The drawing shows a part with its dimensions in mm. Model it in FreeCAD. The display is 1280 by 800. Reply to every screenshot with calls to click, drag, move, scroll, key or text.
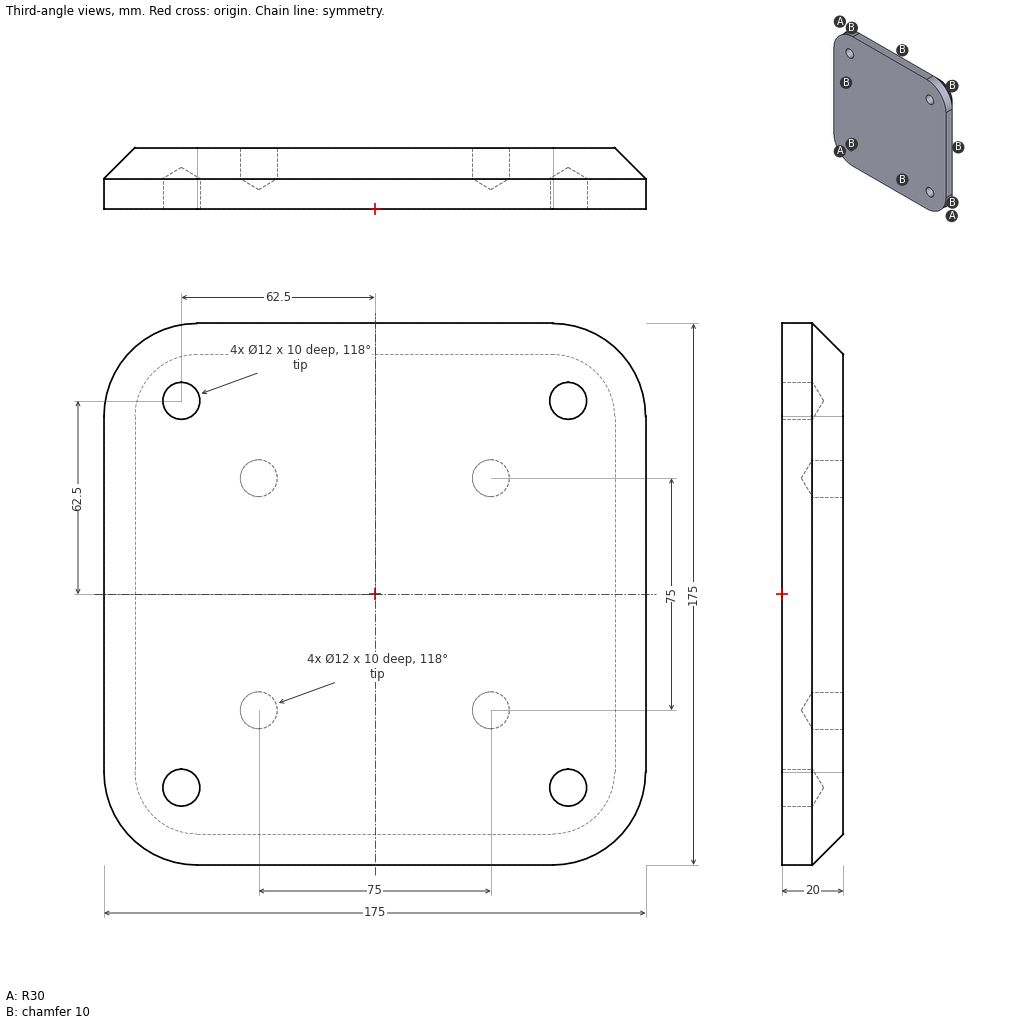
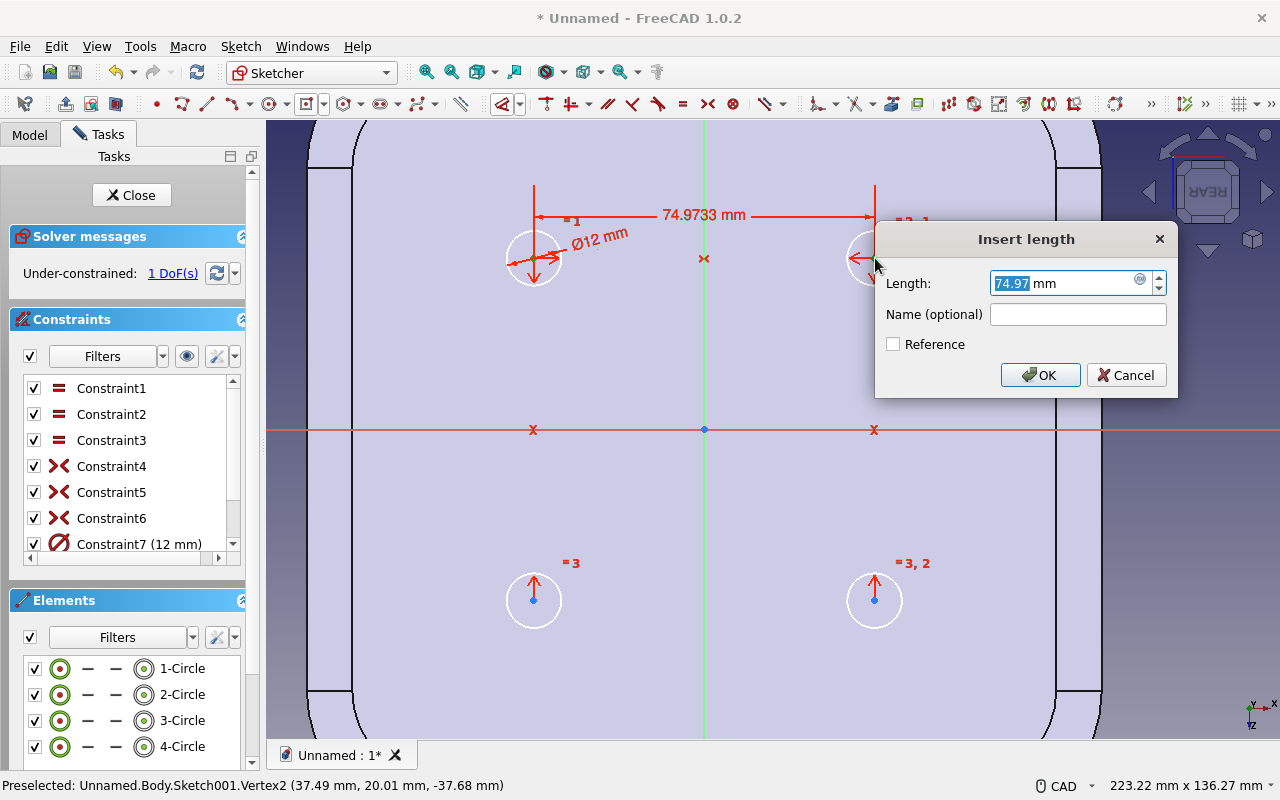
text(75)
key(Return)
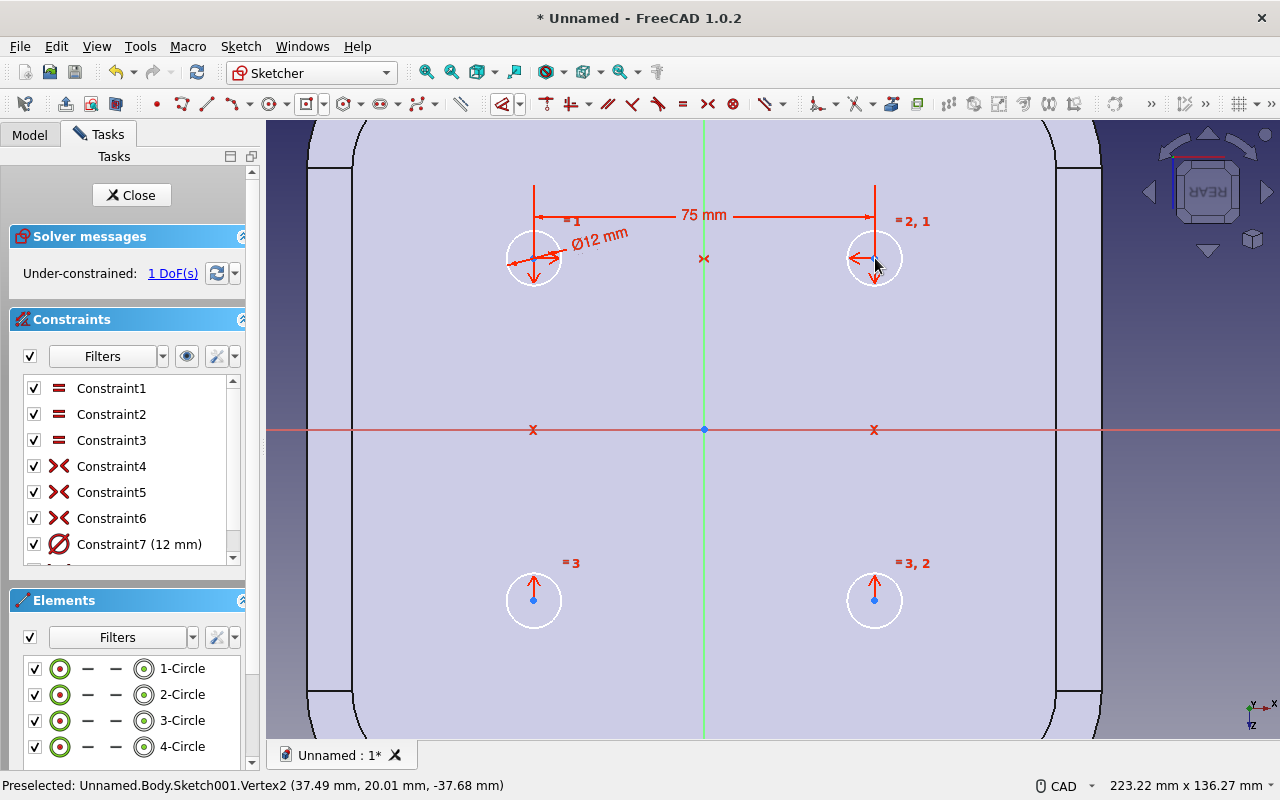
click(875, 258)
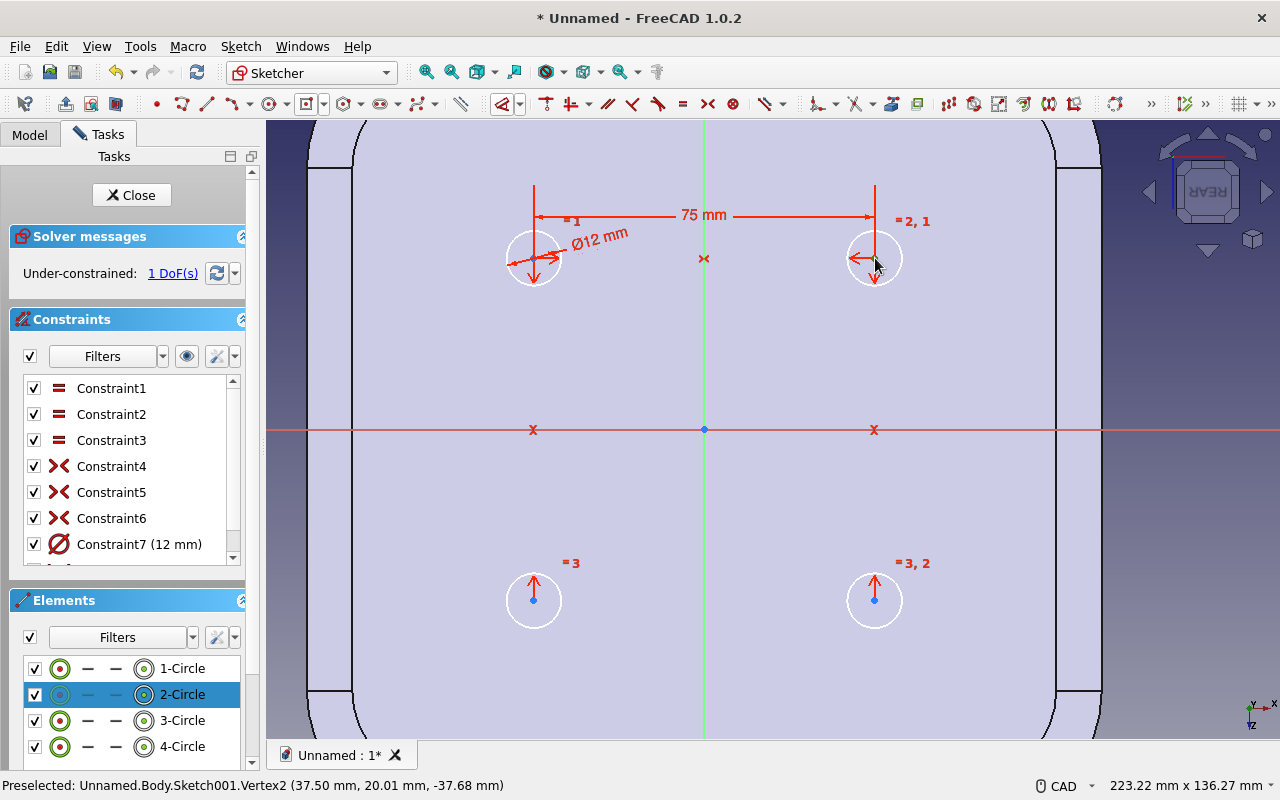
click(875, 601)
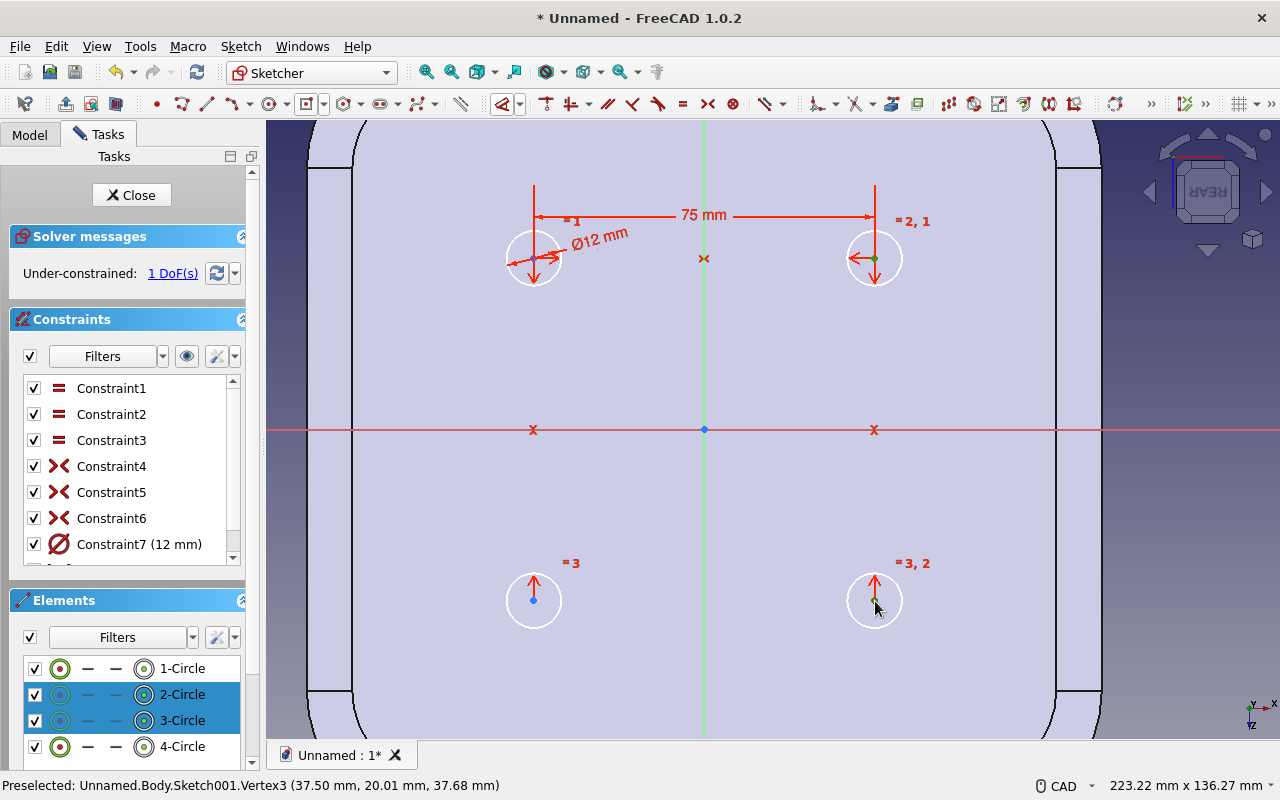
click(520, 104)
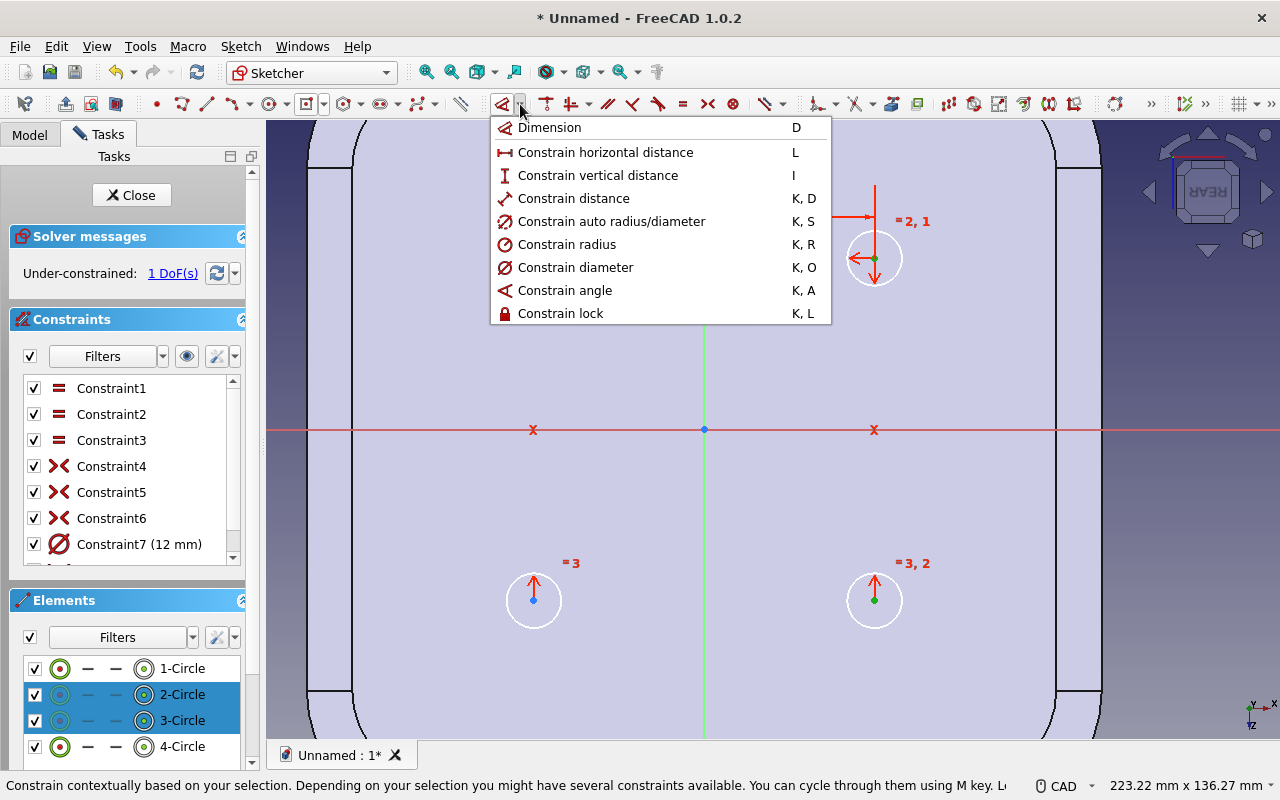
click(661, 176)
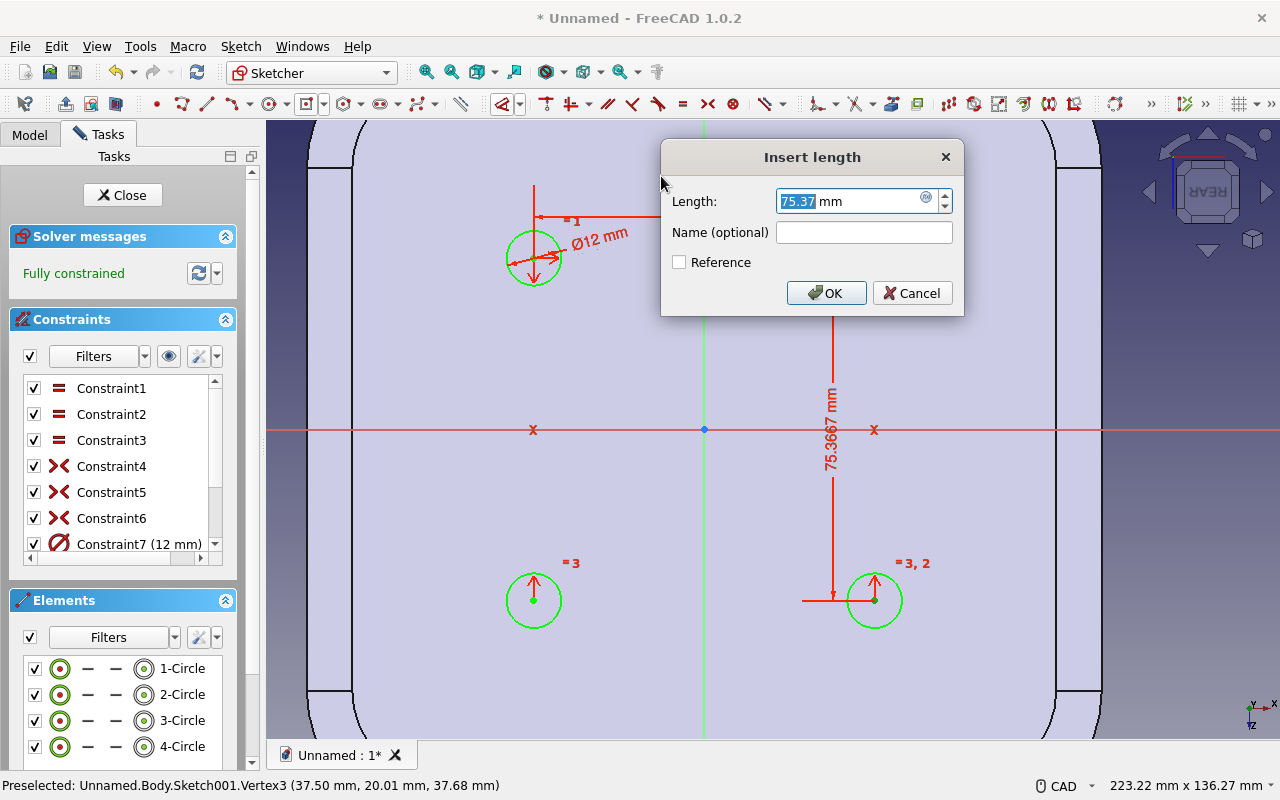
text(75)
key(Return)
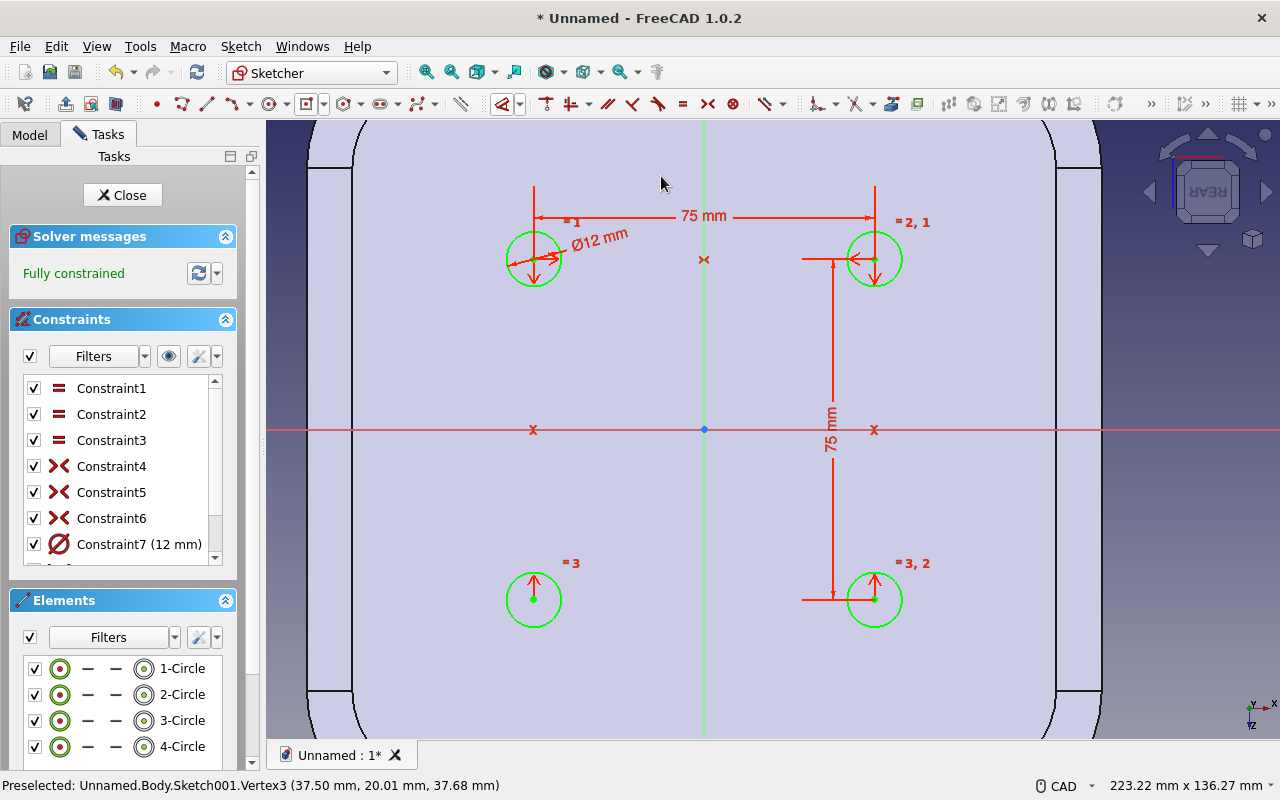
click(123, 195)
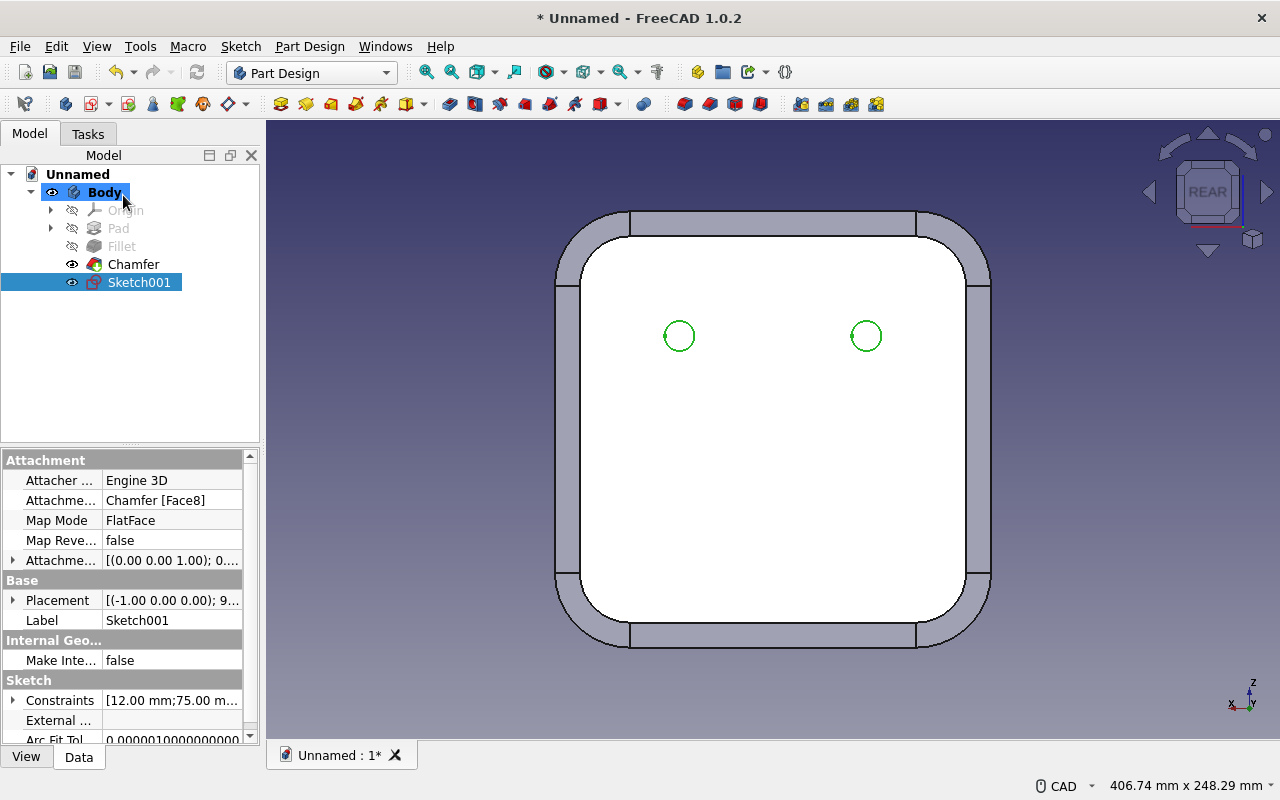
click(475, 104)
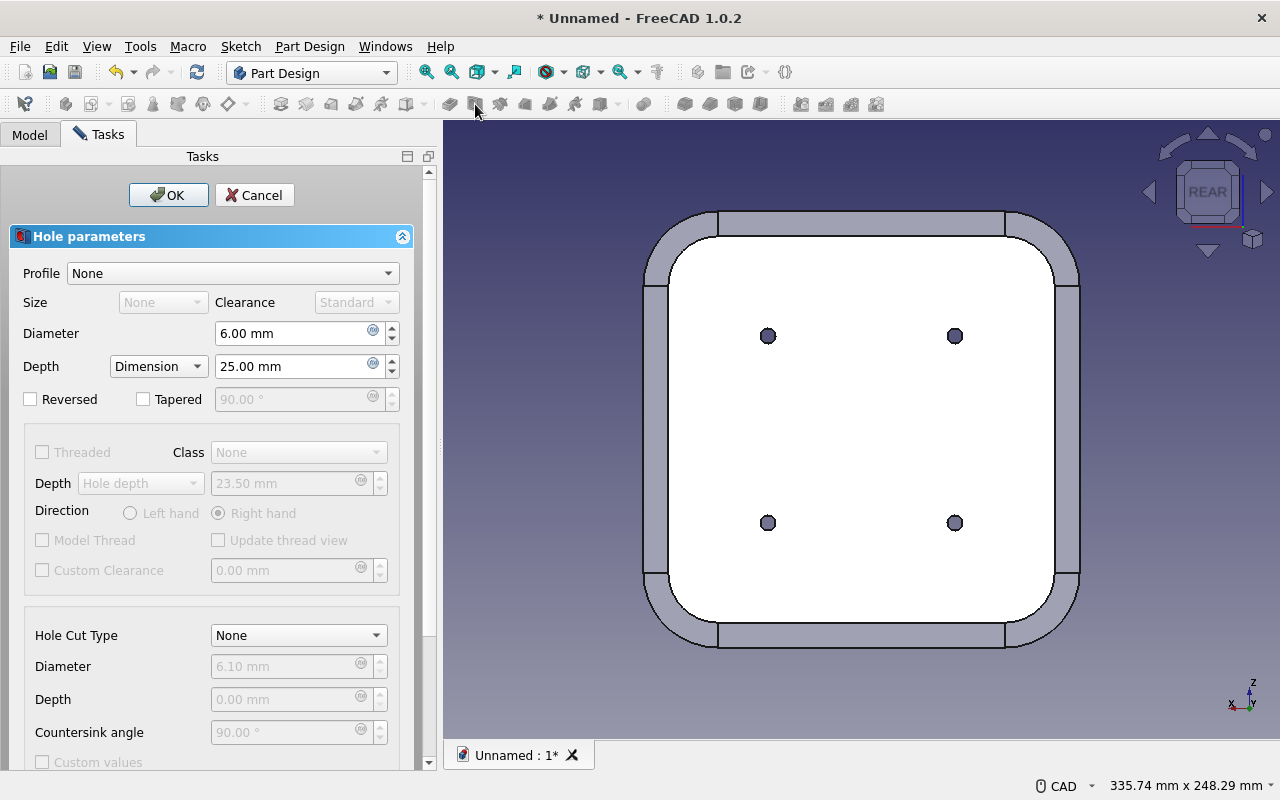
triple_click(300, 334)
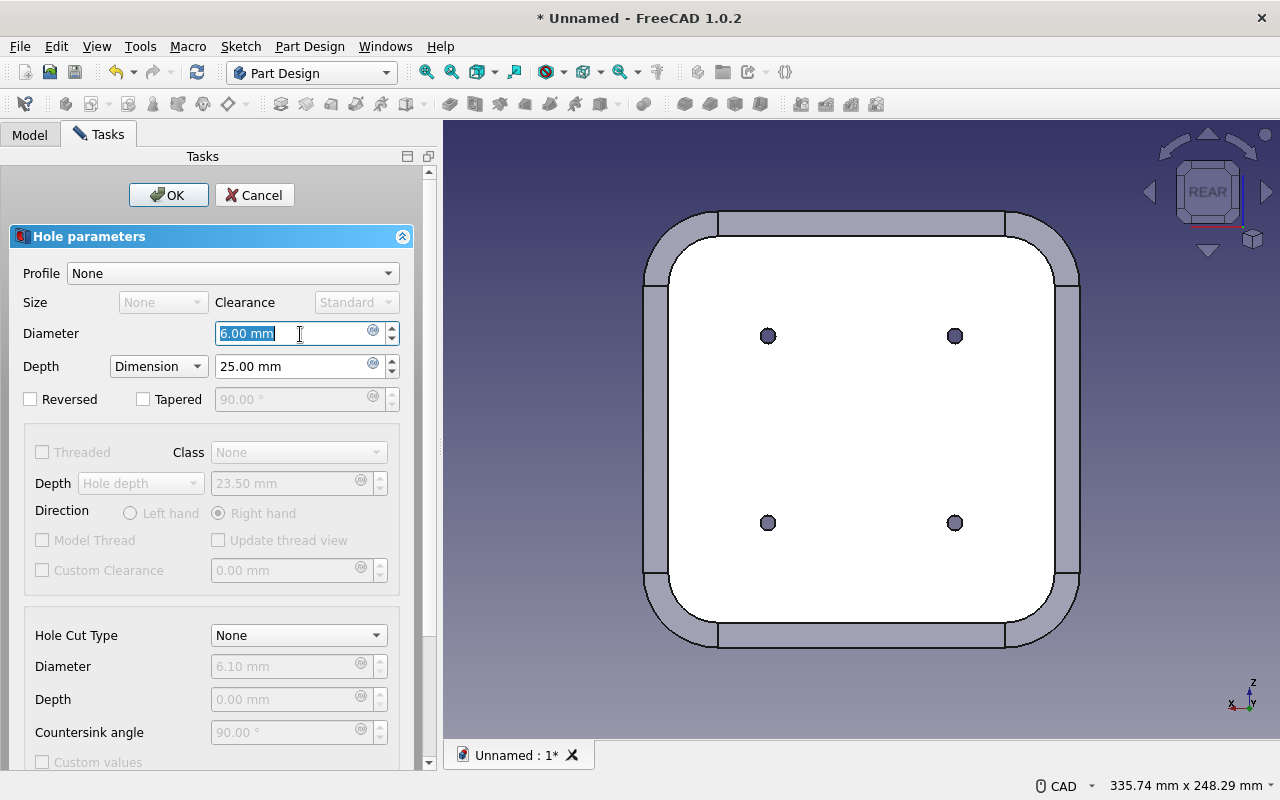
text(12)
key(Tab)